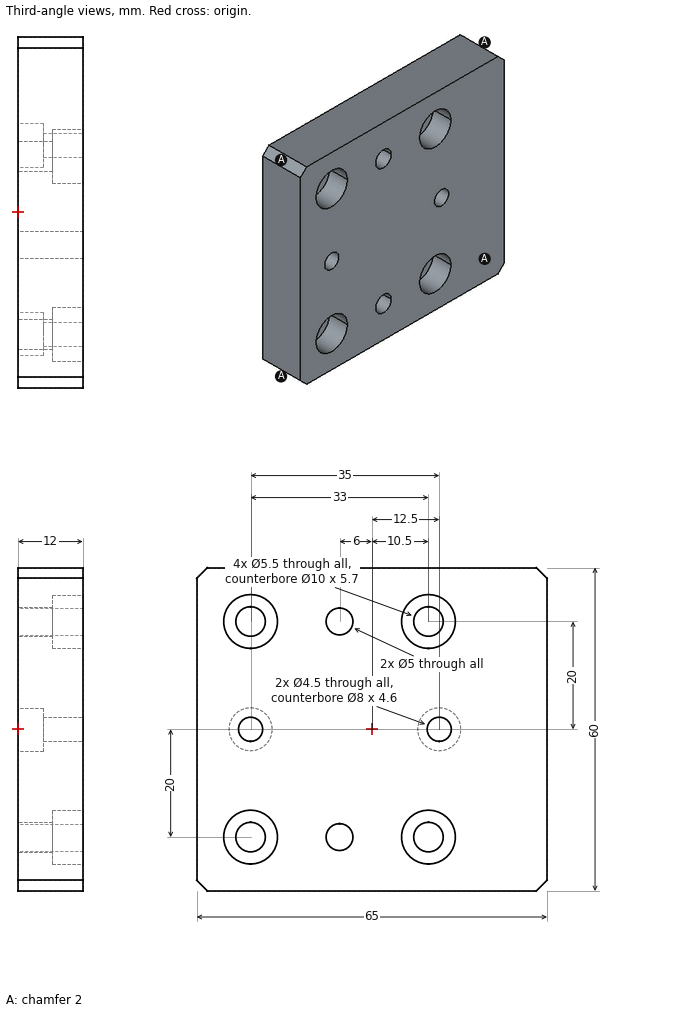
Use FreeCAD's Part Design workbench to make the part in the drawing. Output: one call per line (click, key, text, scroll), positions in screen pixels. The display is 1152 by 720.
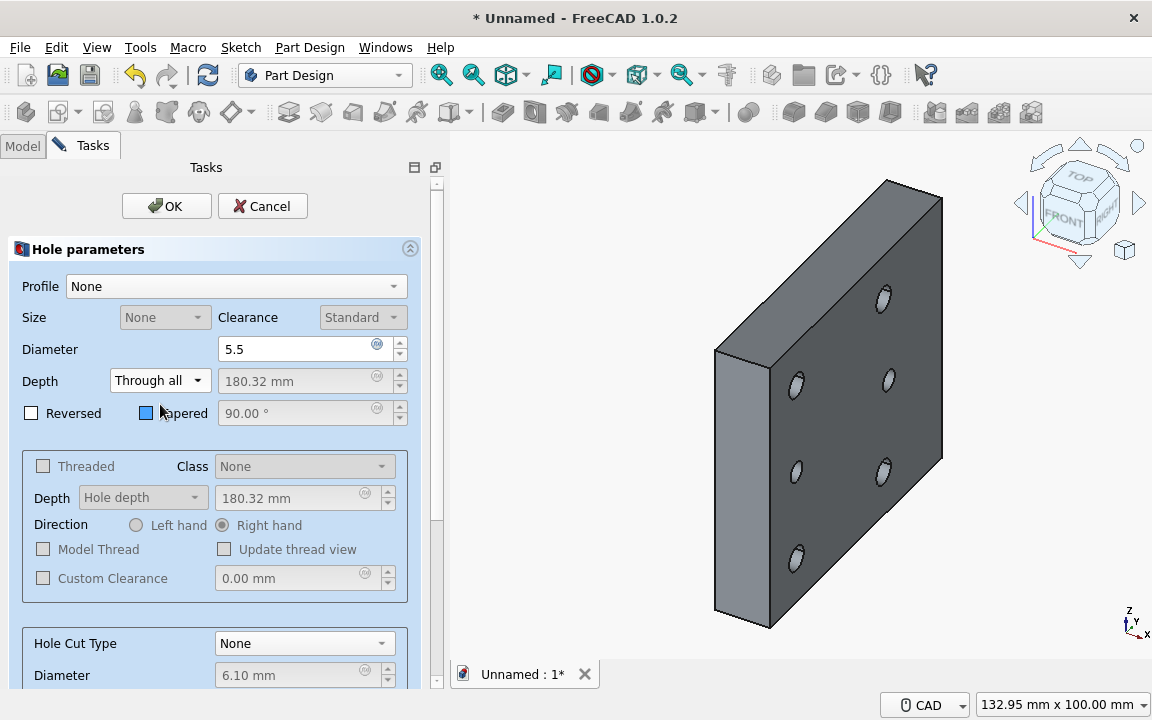
click(306, 644)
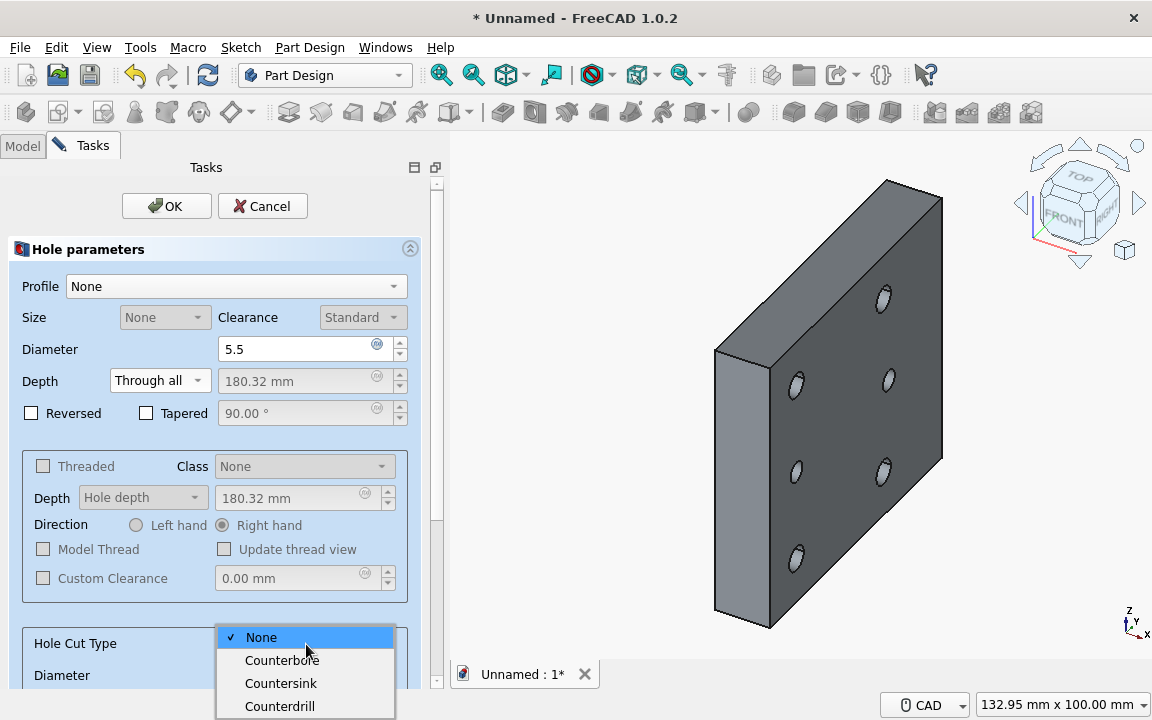
click(304, 660)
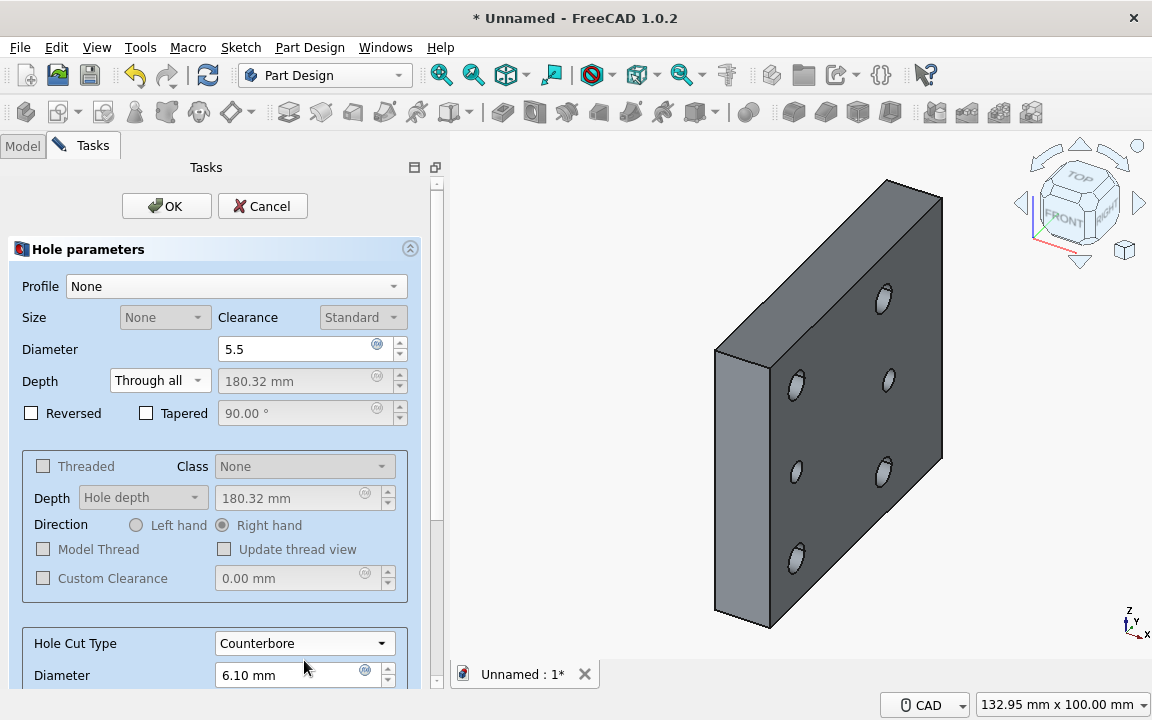
triple_click(298, 675)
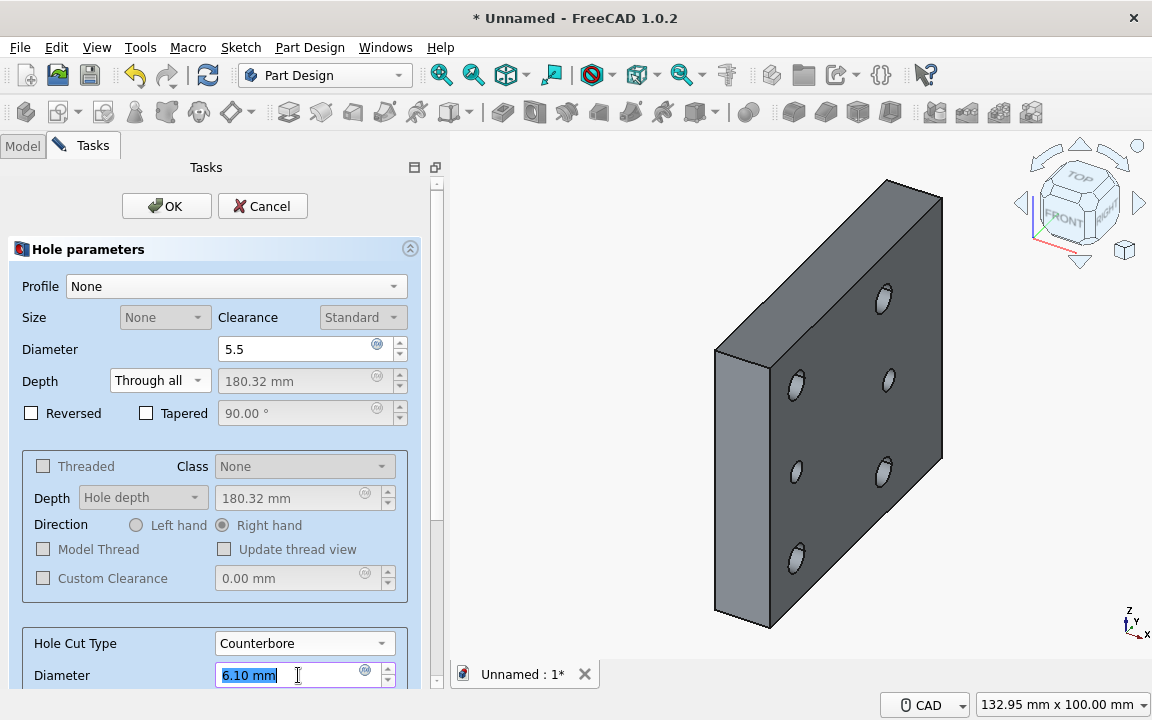
text(10)
key(Tab)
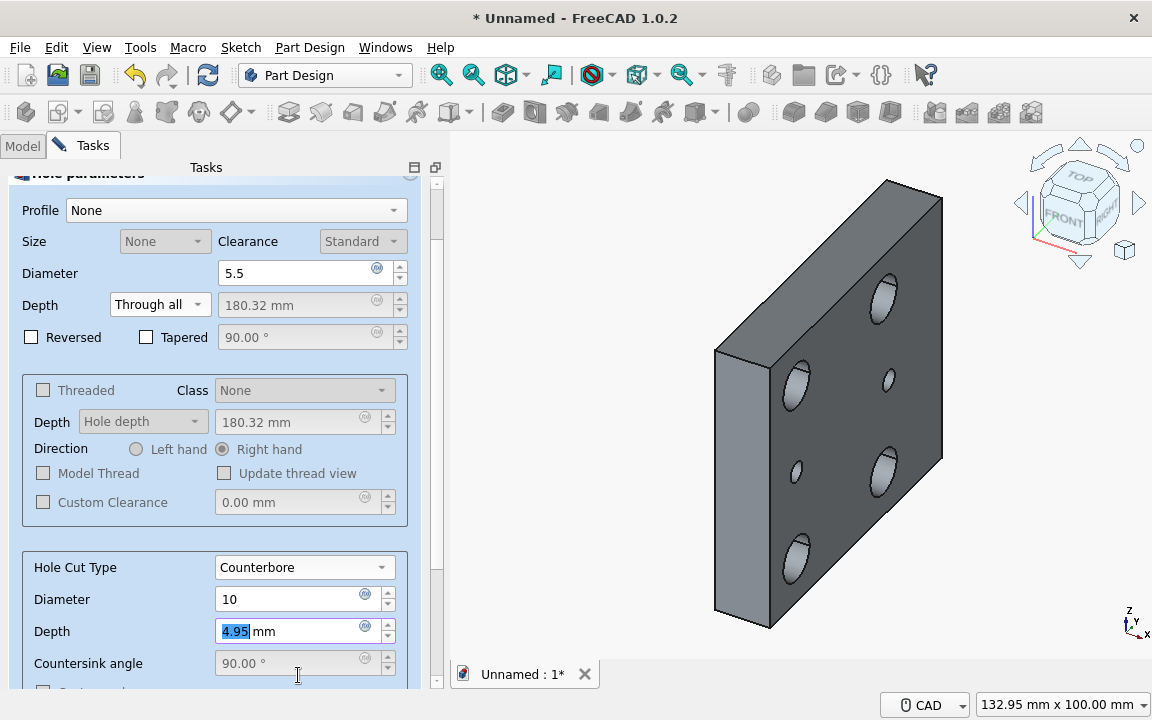
text(5.7)
key(Tab)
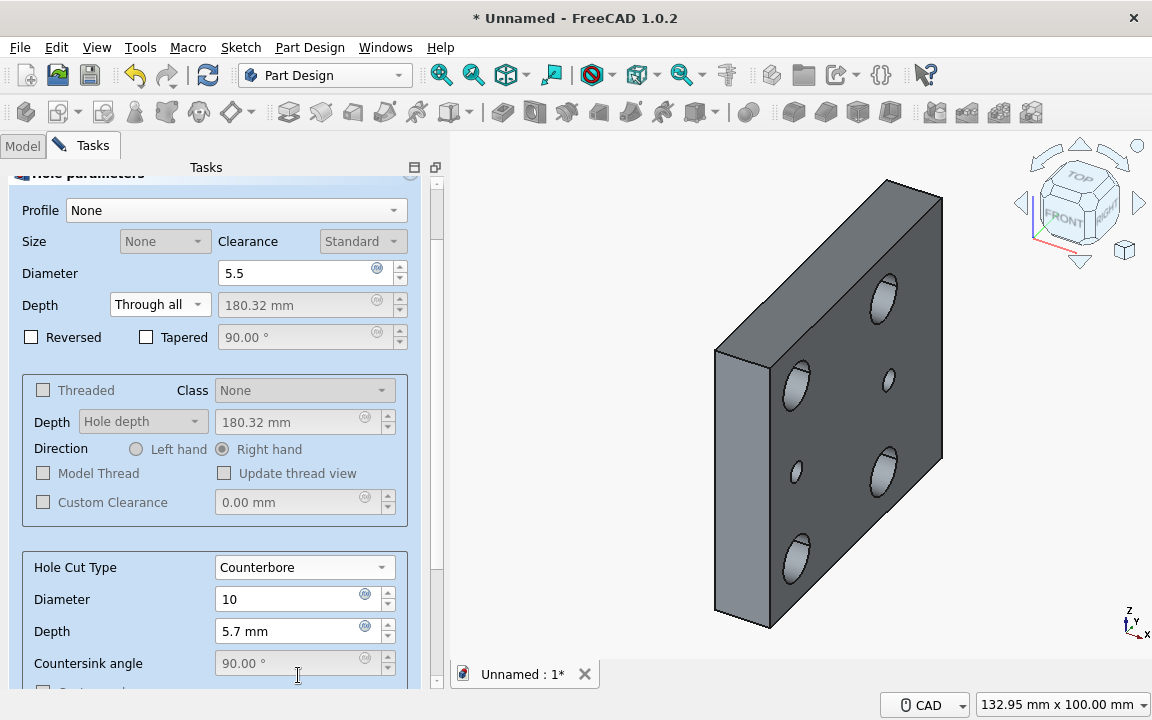
scroll(437, 432, up, 3)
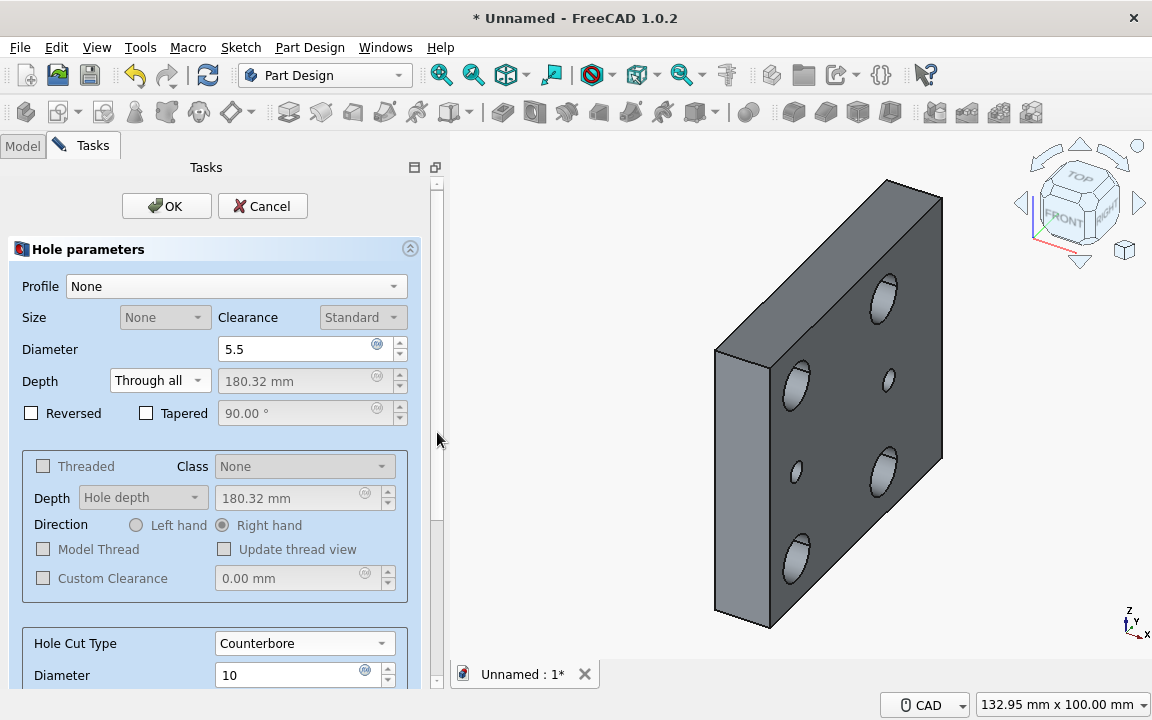
click(167, 206)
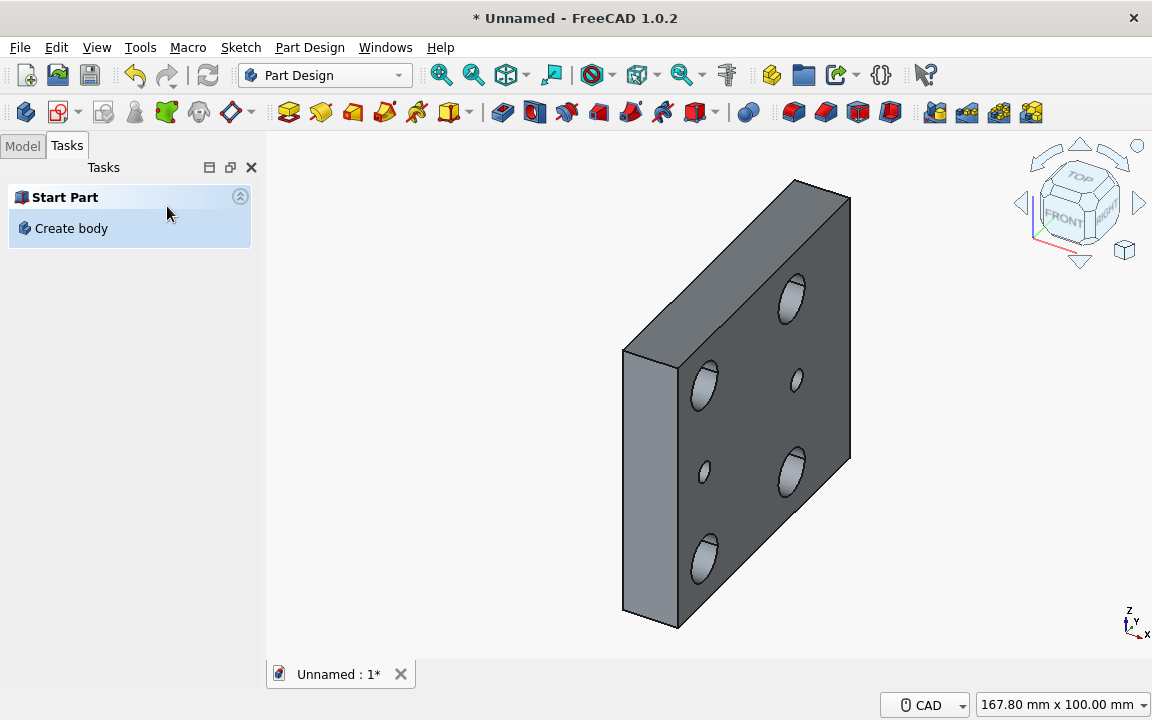
click(651, 359)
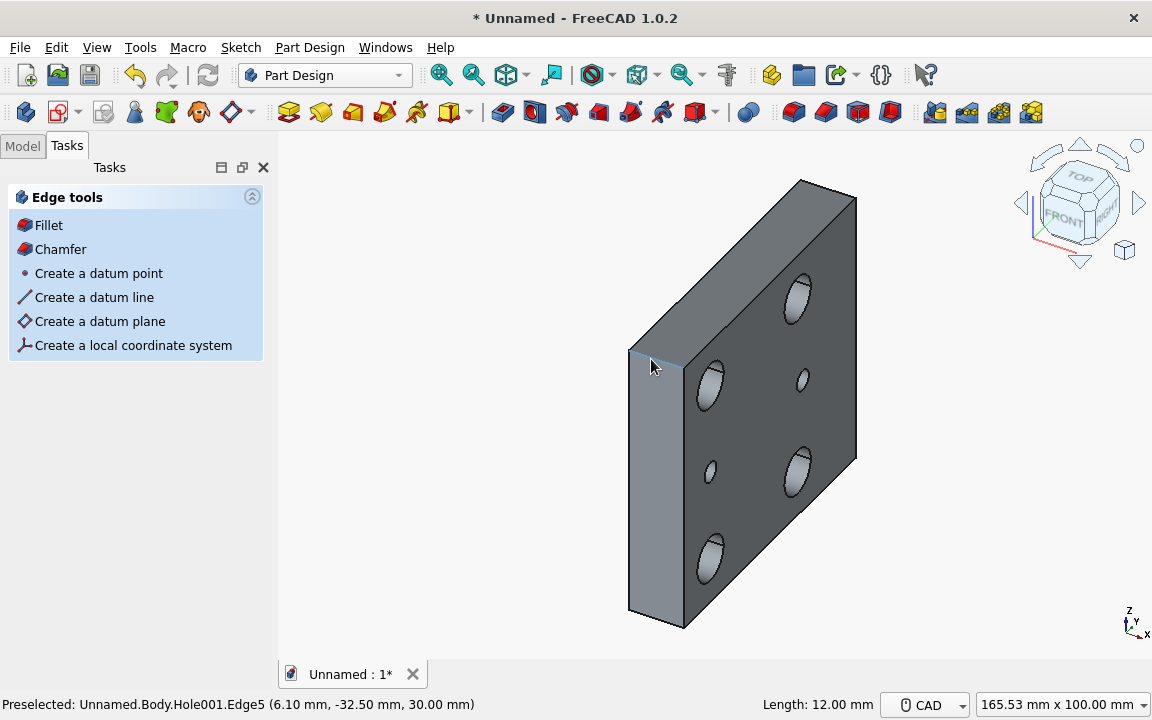
key(0)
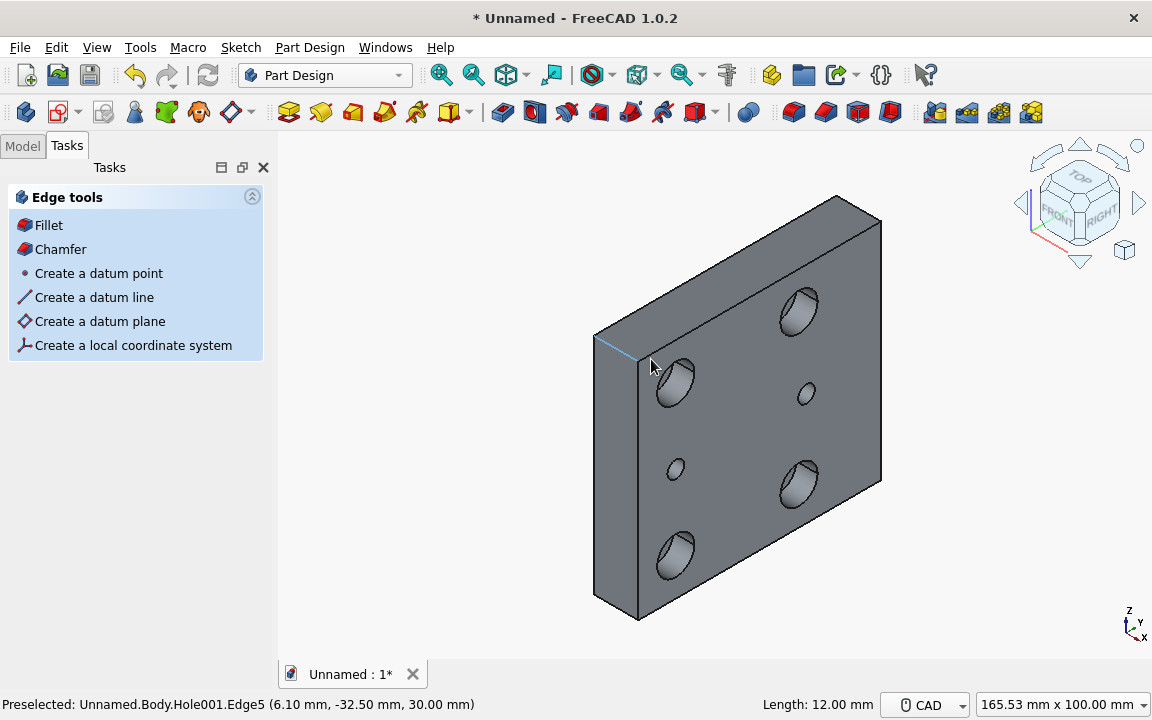
key(2)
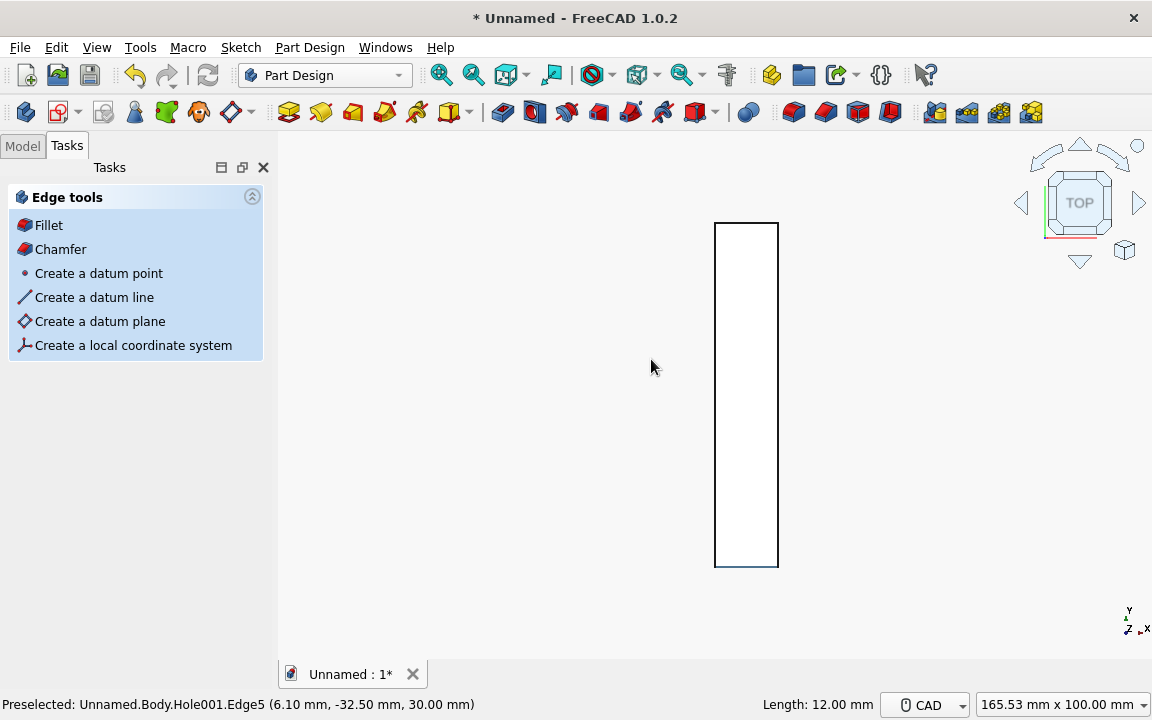
click(747, 222, ctrl)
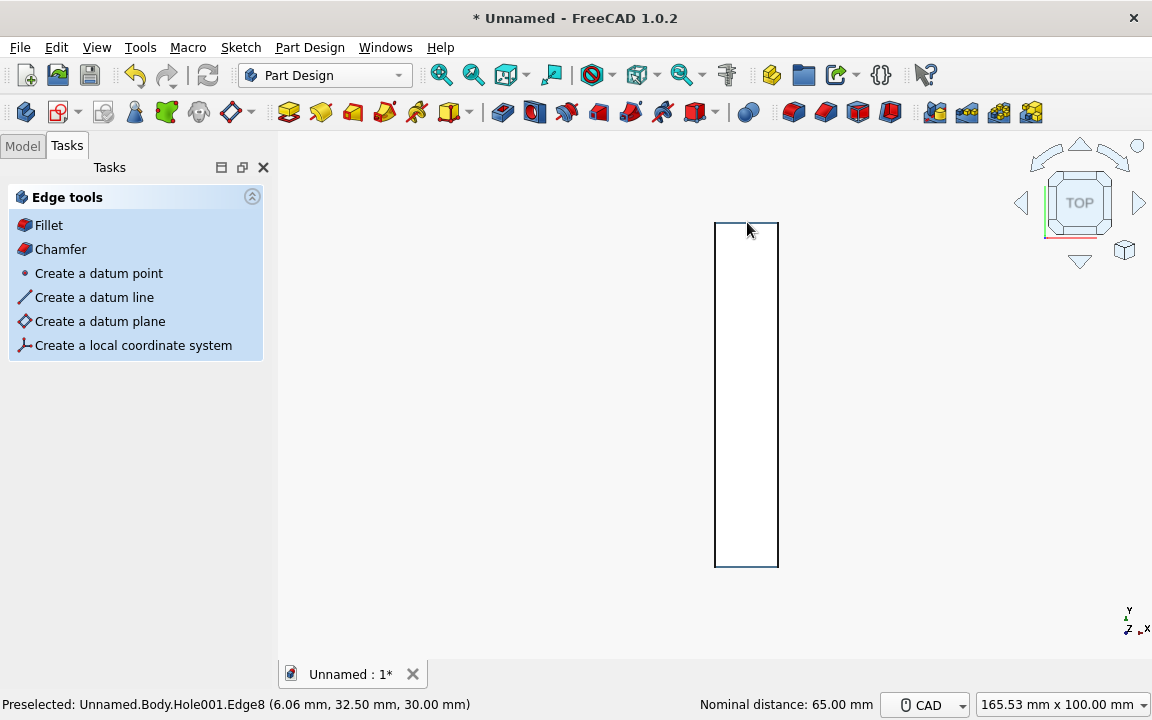
key(1)